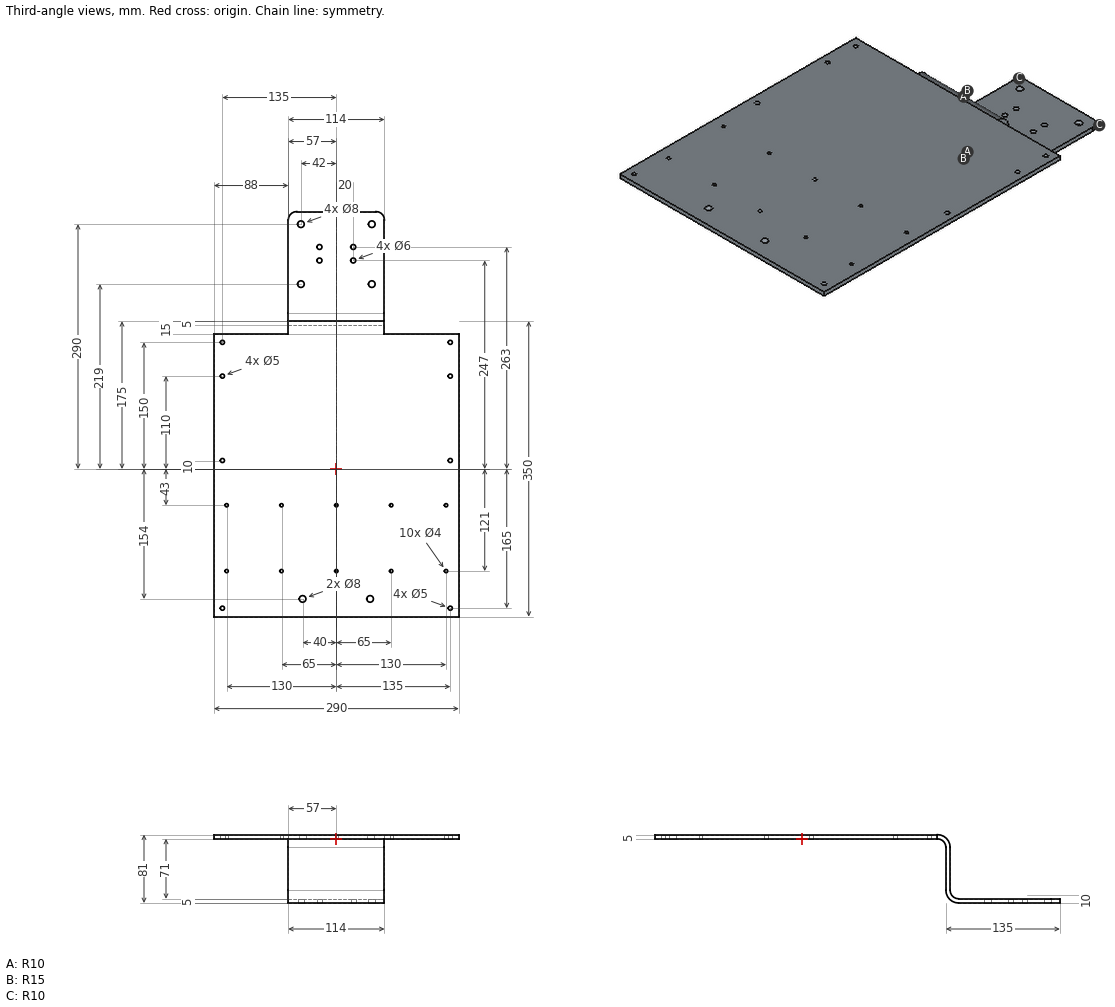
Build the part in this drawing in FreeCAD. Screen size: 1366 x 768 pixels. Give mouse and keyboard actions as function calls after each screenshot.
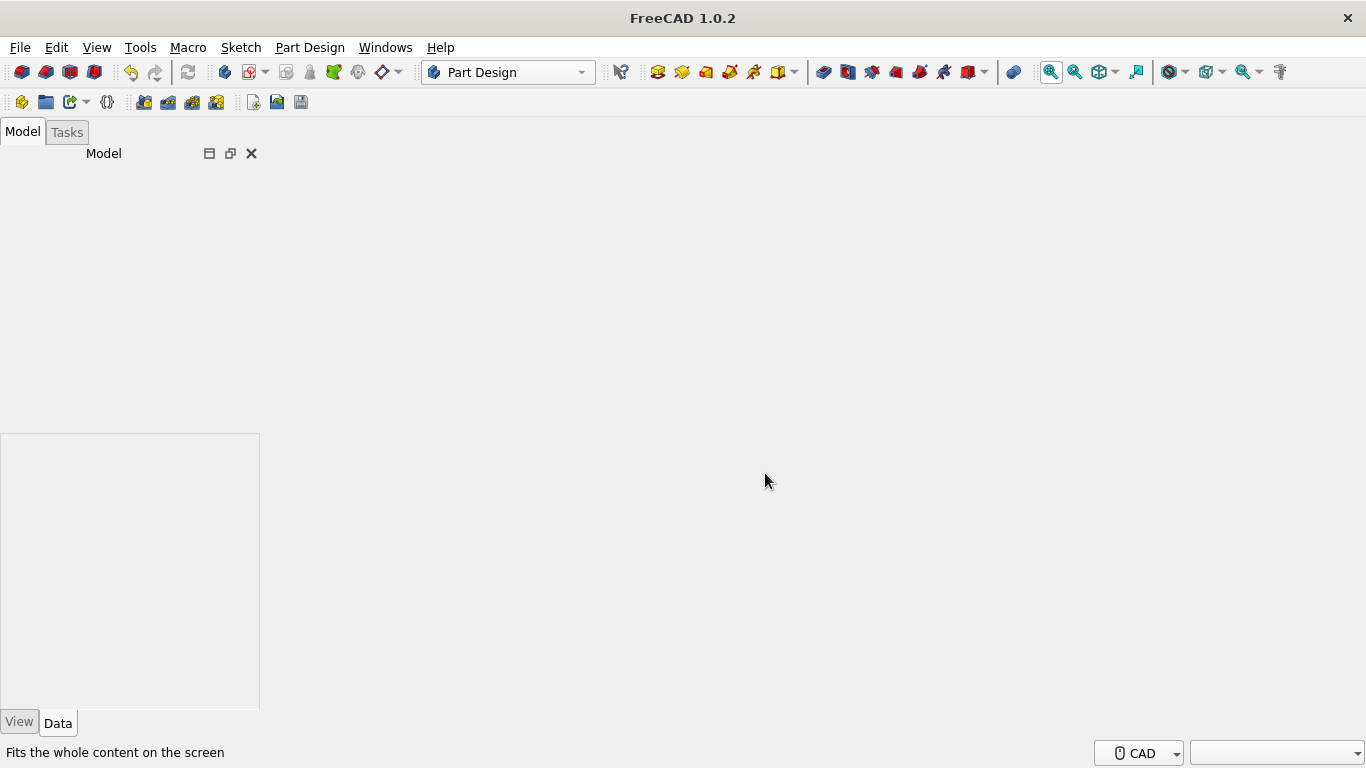
click(254, 102)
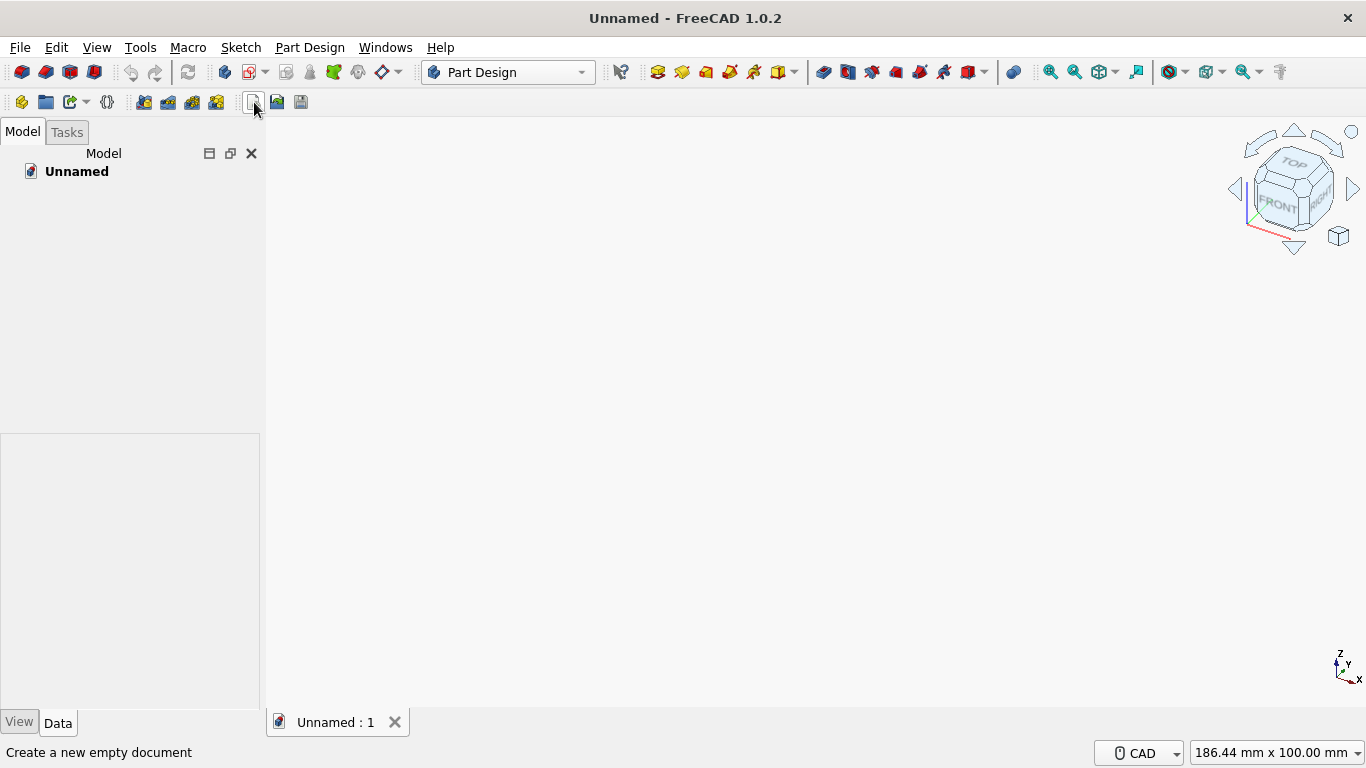
click(250, 72)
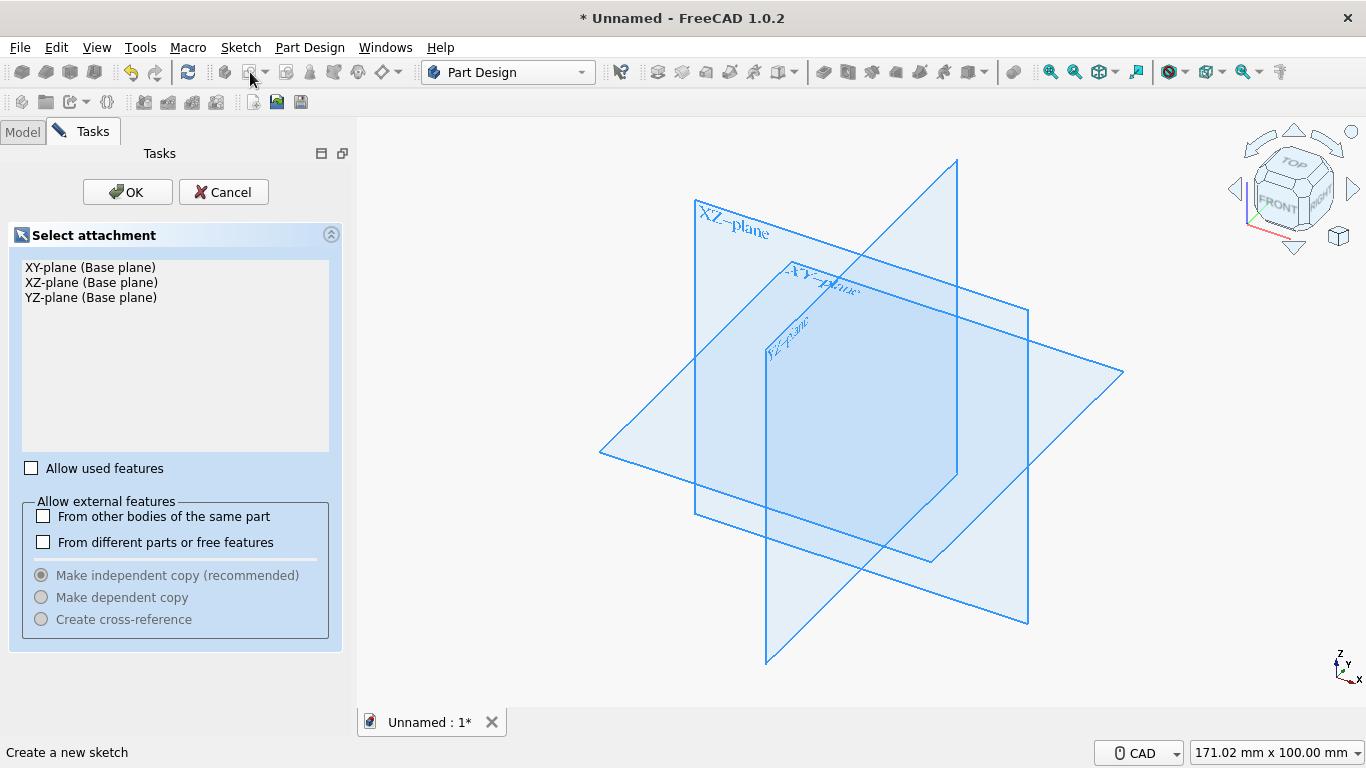
click(82, 268)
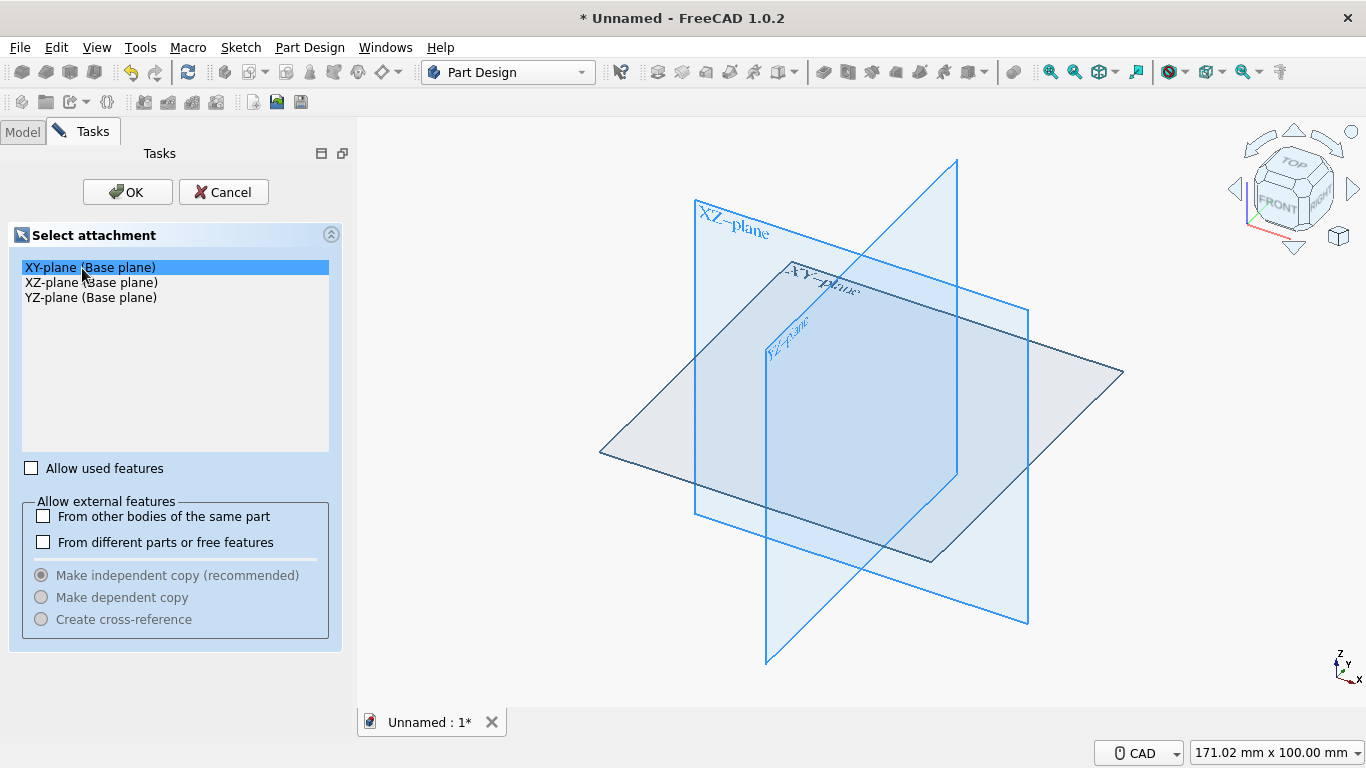
click(128, 192)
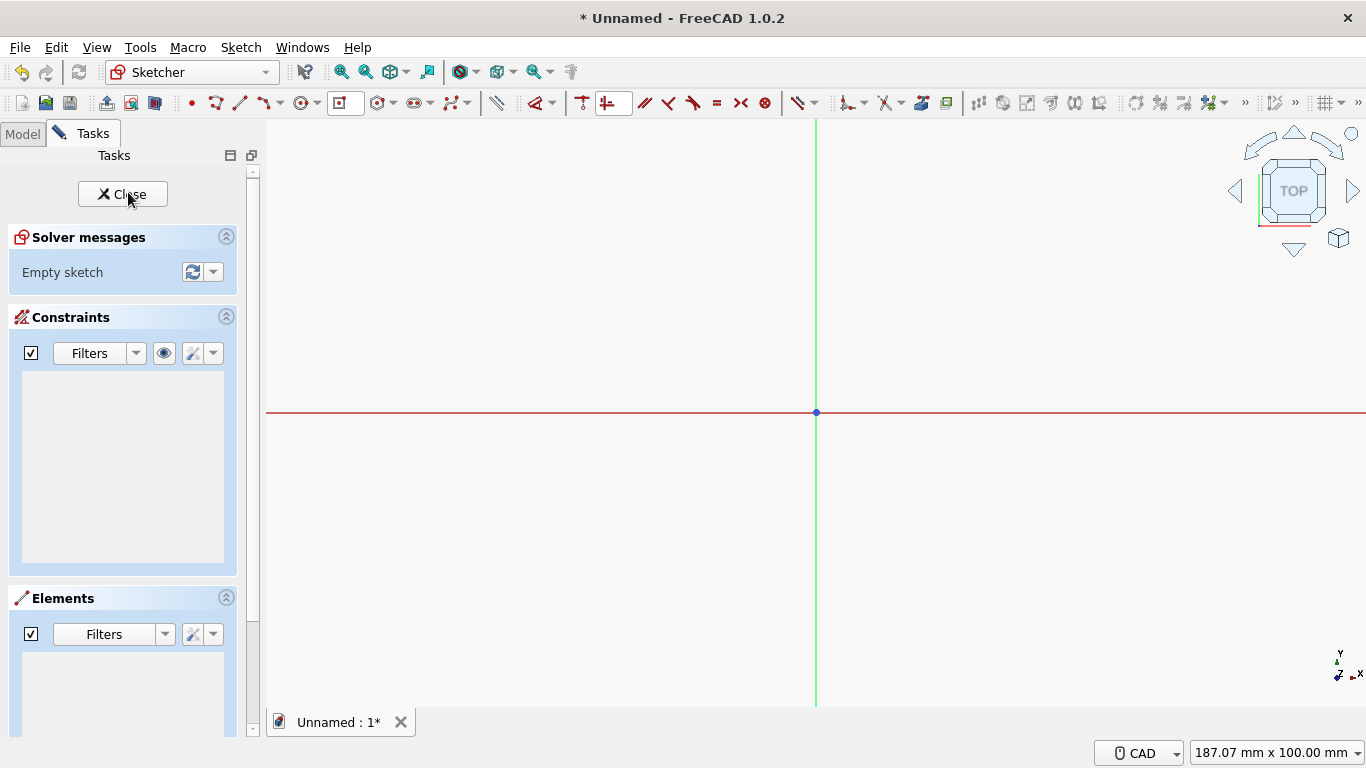
scroll(734, 413, down, 9)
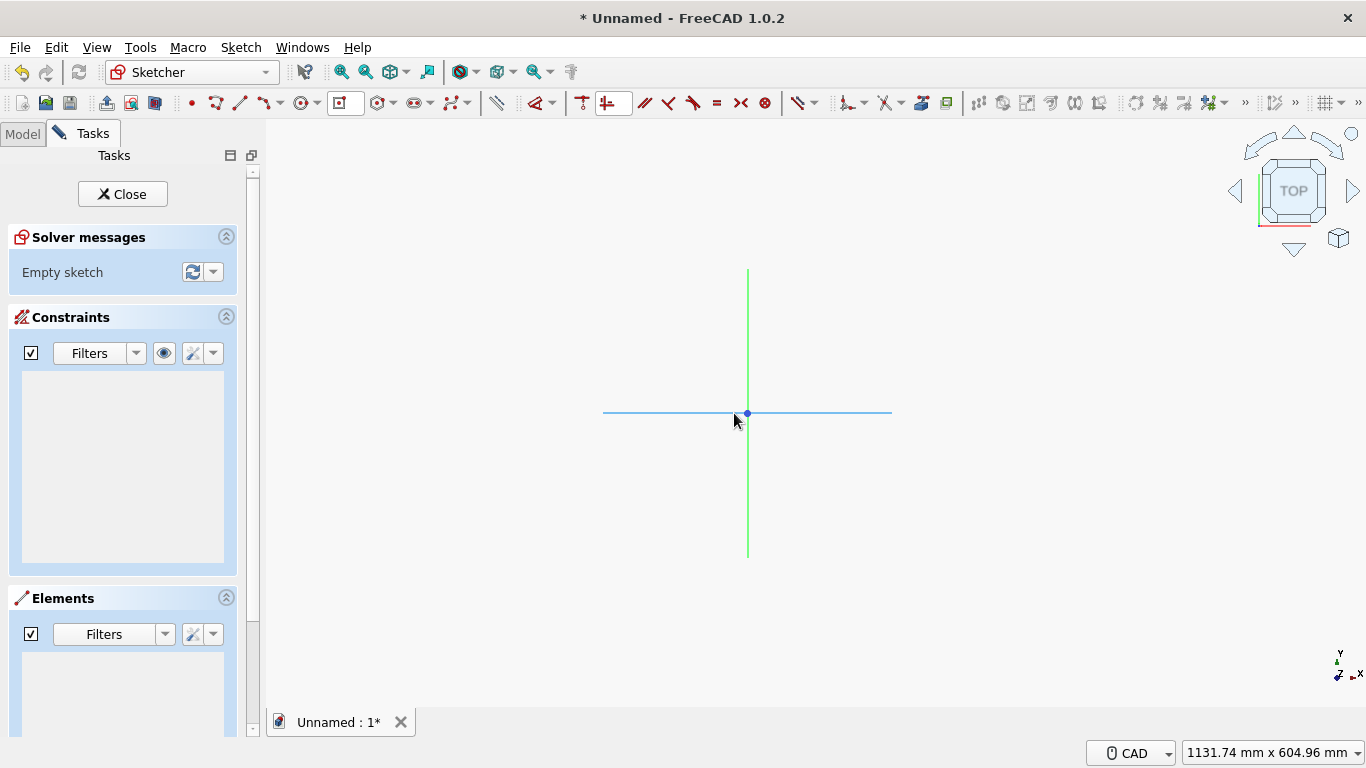
click(340, 104)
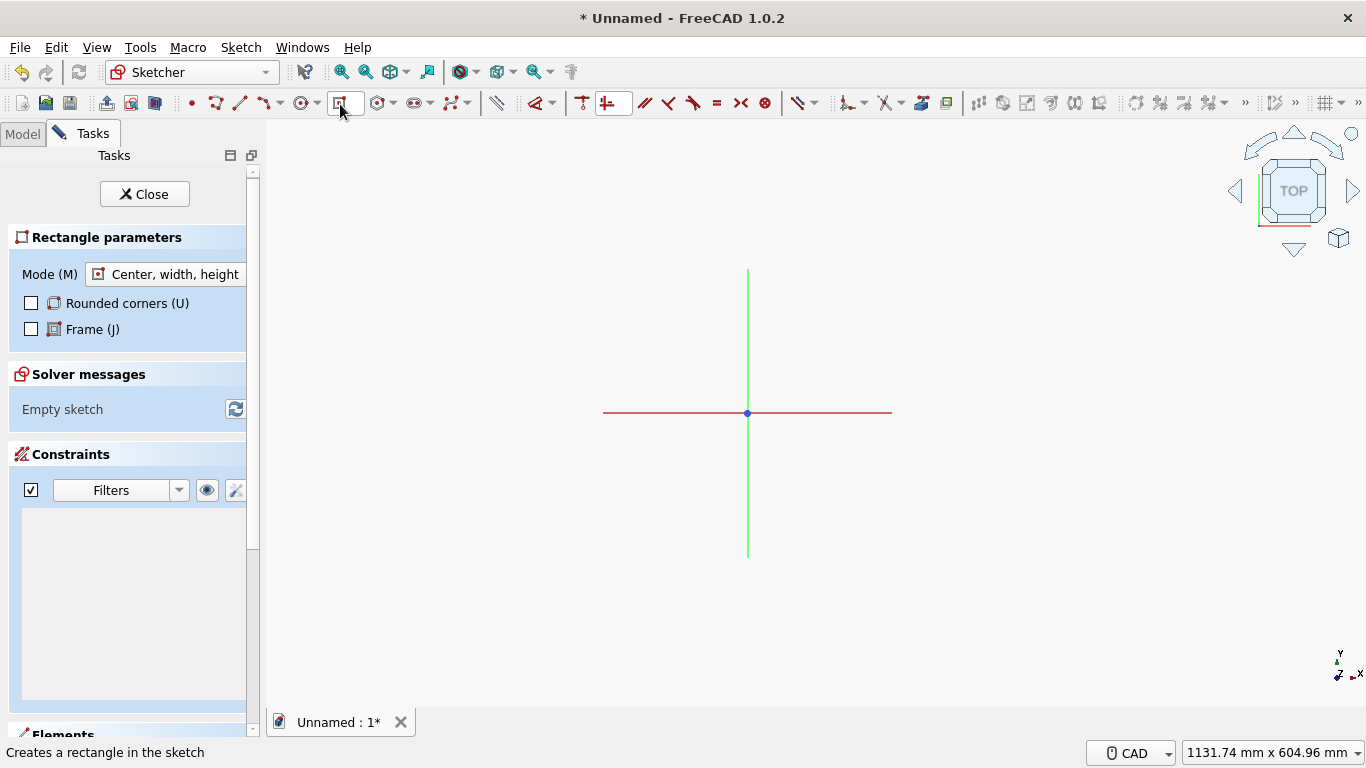
click(748, 413)
click(889, 243)
key(Escape)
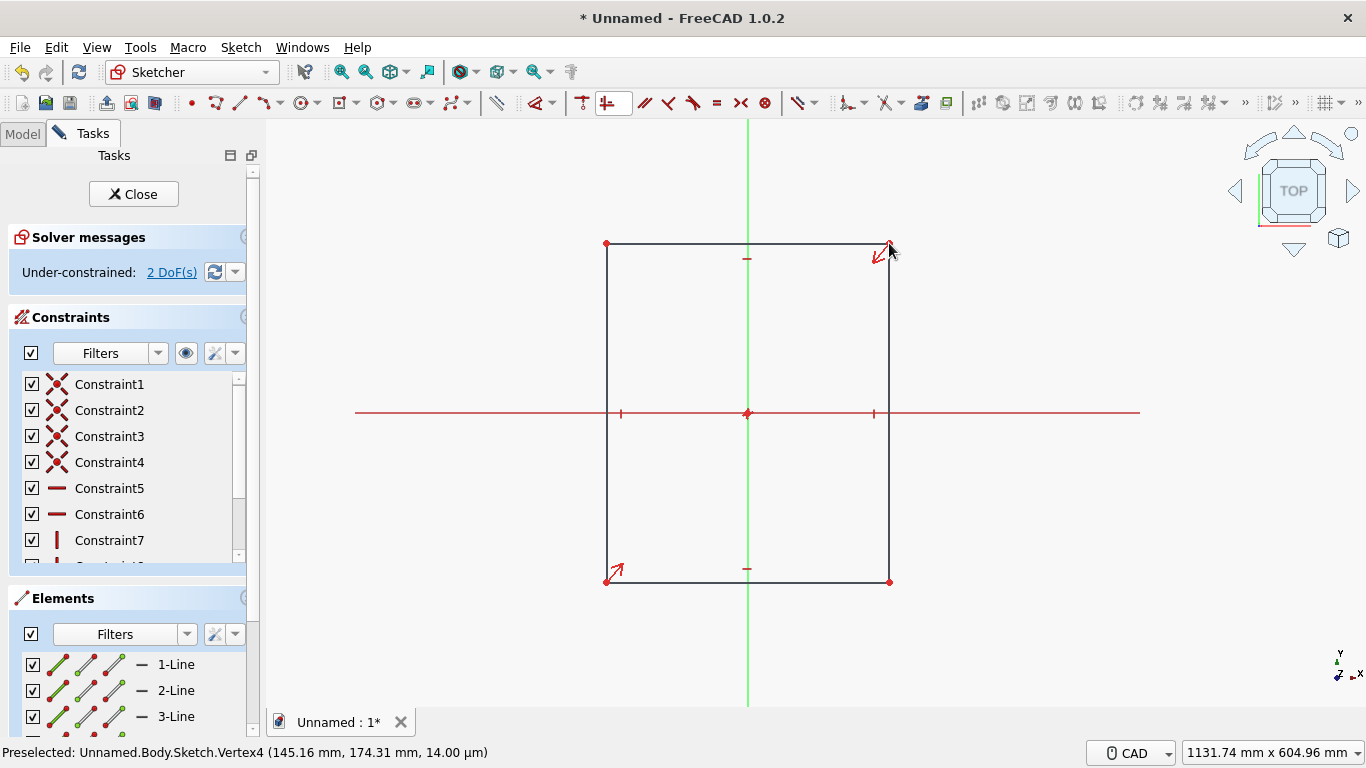
click(536, 104)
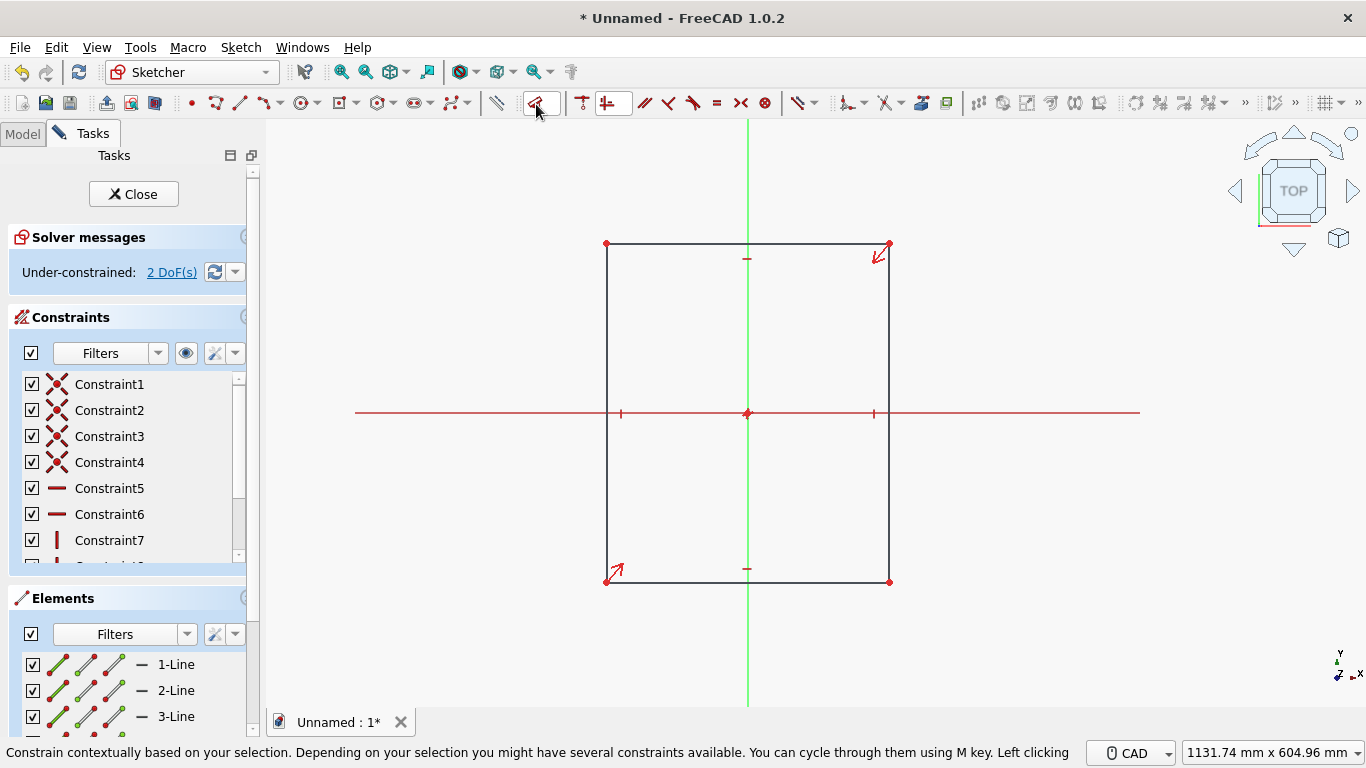
click(691, 583)
click(683, 617)